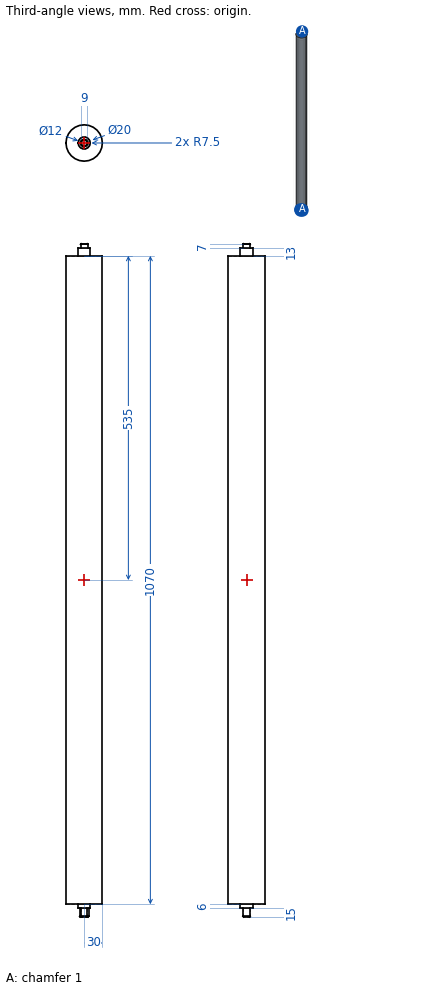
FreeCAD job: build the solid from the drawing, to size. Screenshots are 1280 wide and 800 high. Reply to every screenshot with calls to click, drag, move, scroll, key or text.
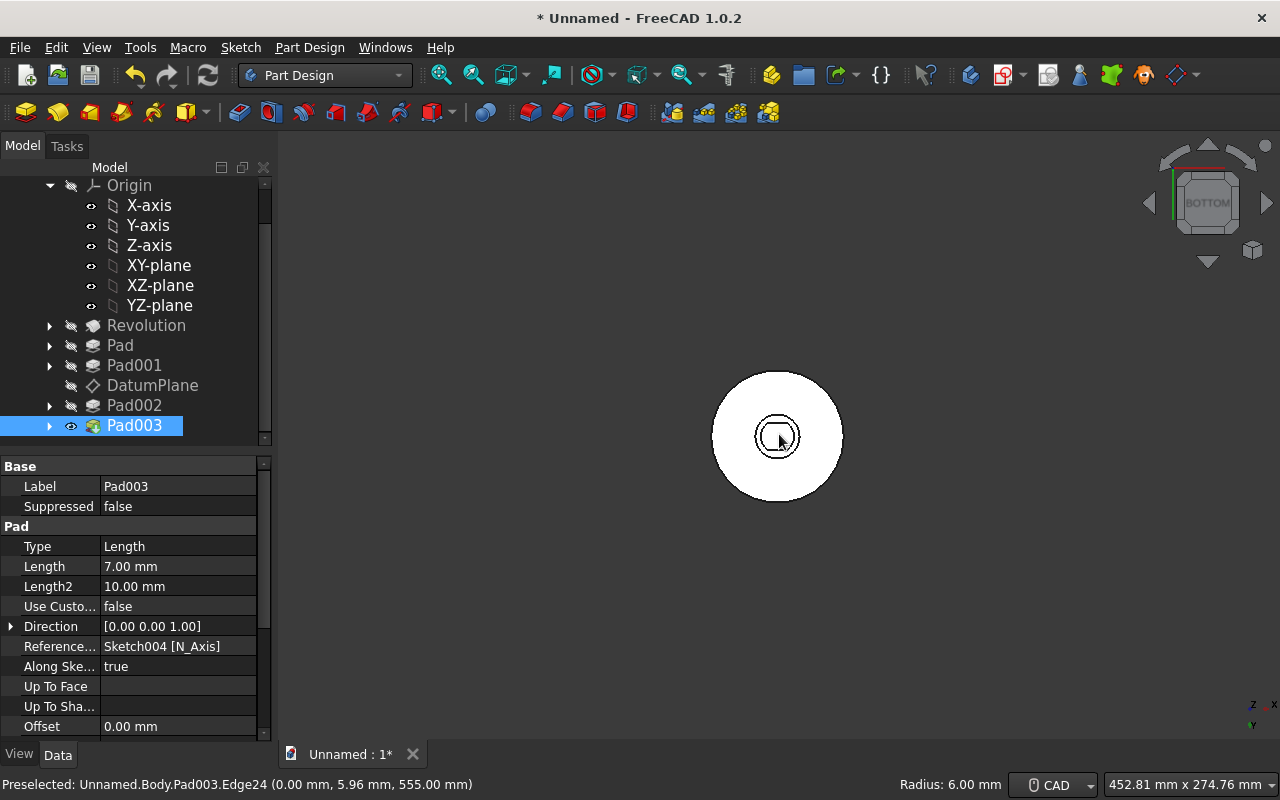
click(777, 436, ctrl)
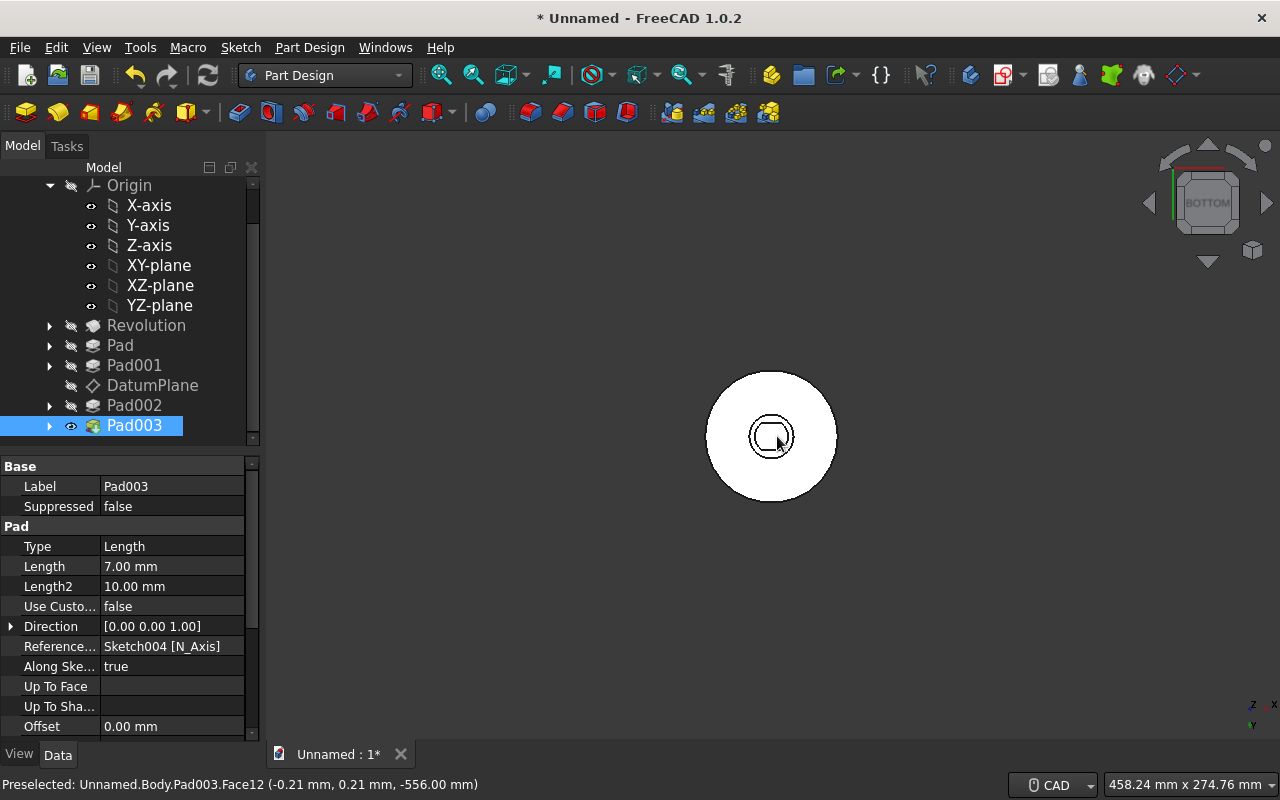
click(564, 112)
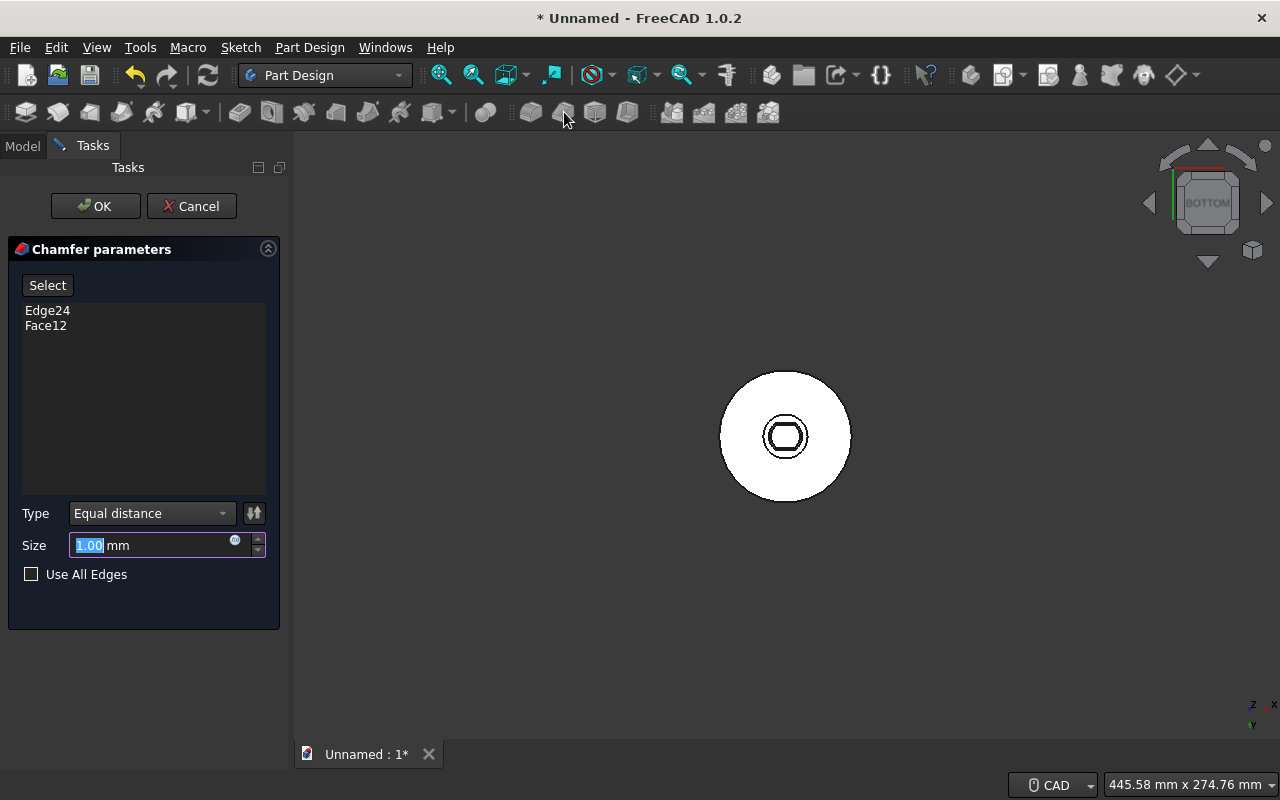
text(1)
key(Tab)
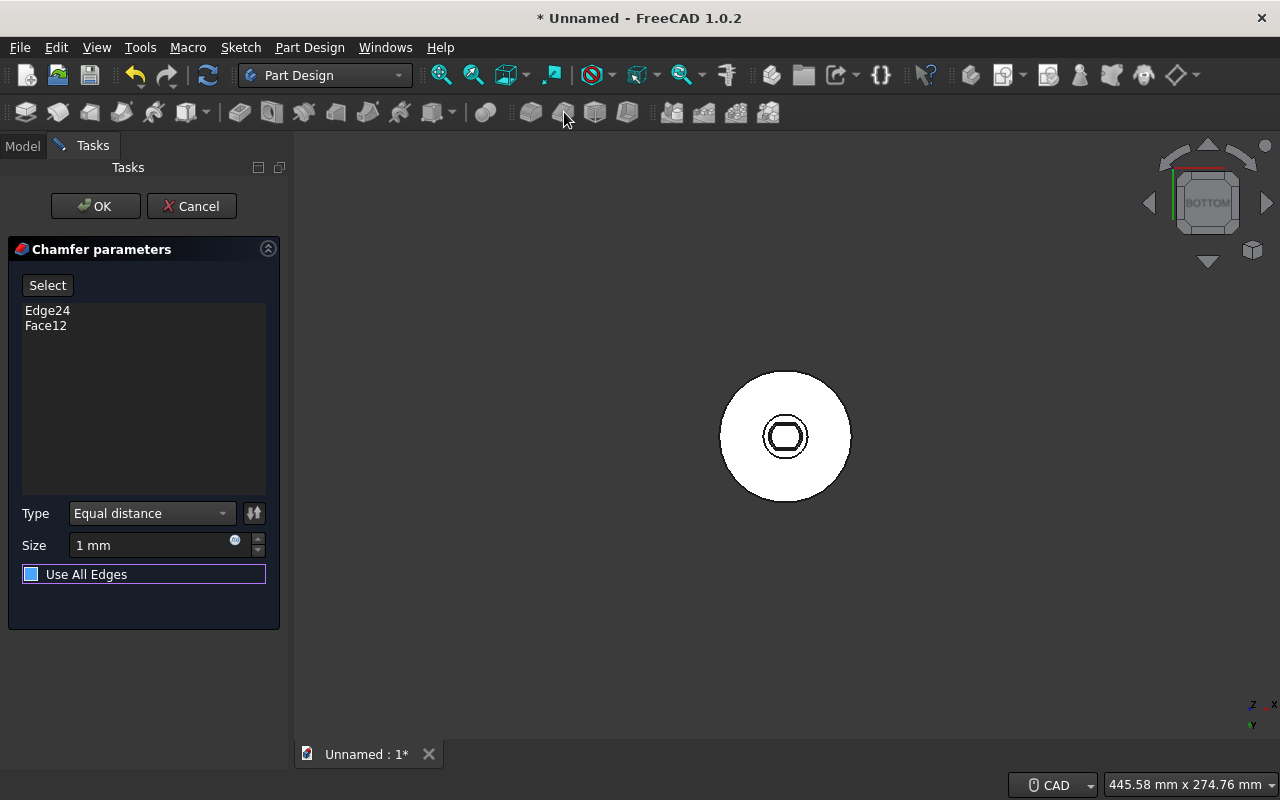
click(96, 206)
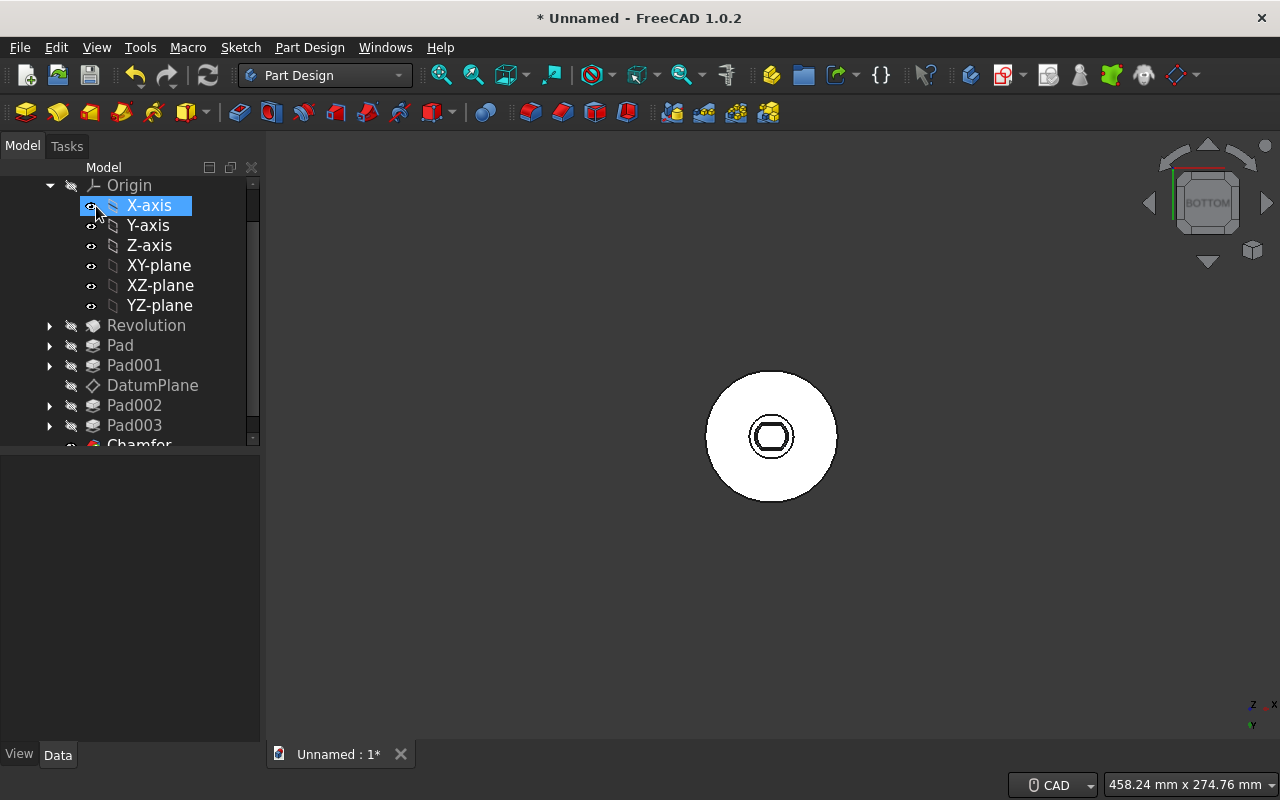
key(0)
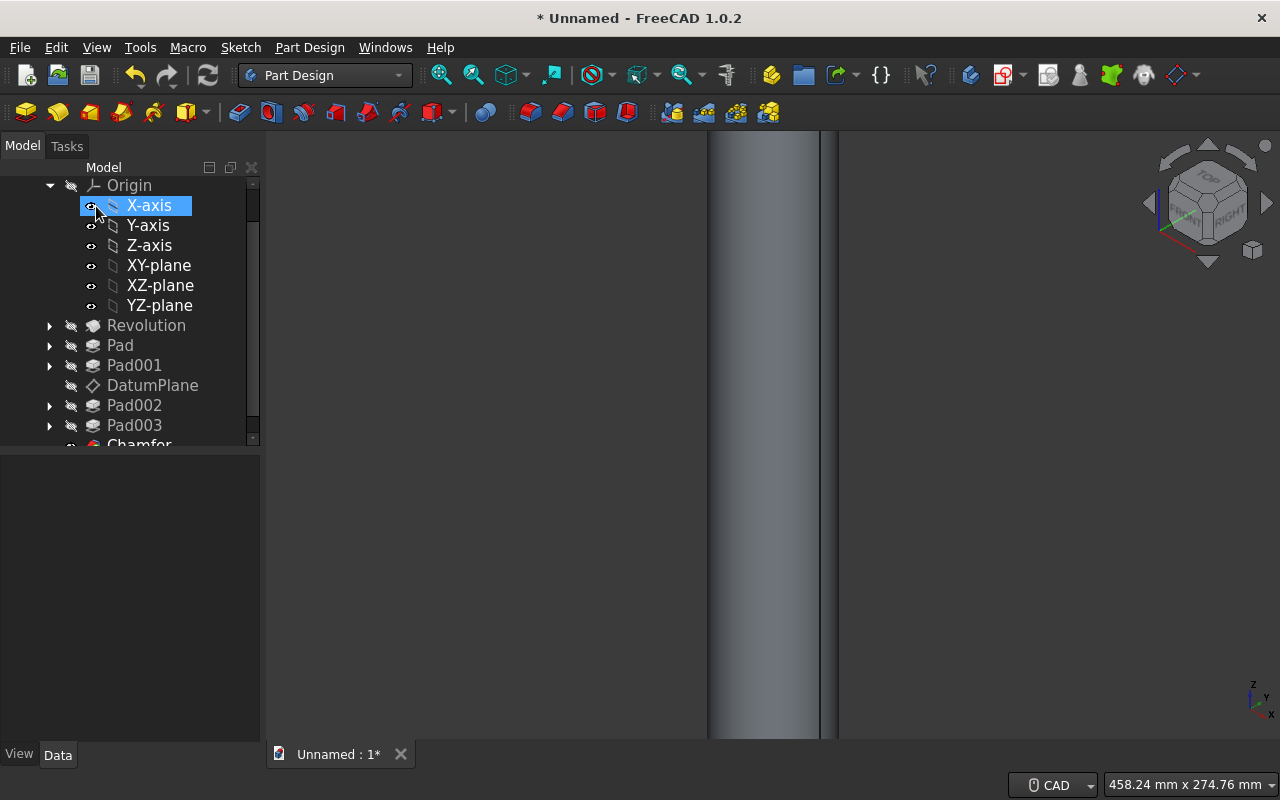
key(v)
key(f)